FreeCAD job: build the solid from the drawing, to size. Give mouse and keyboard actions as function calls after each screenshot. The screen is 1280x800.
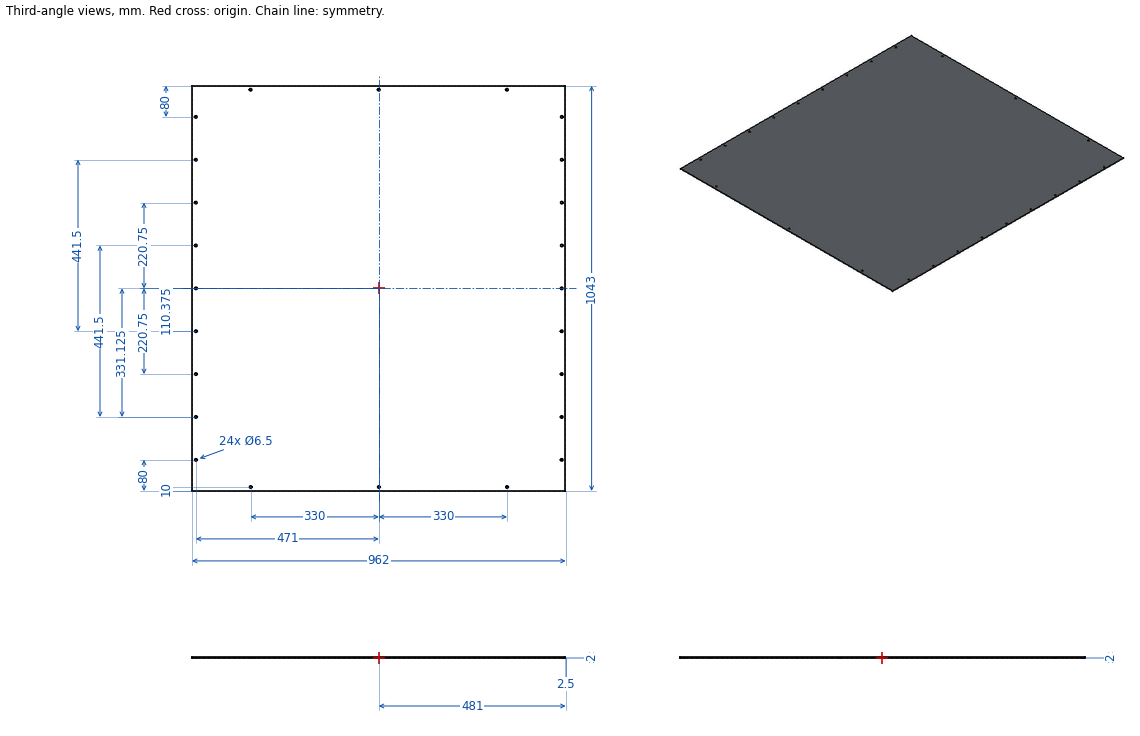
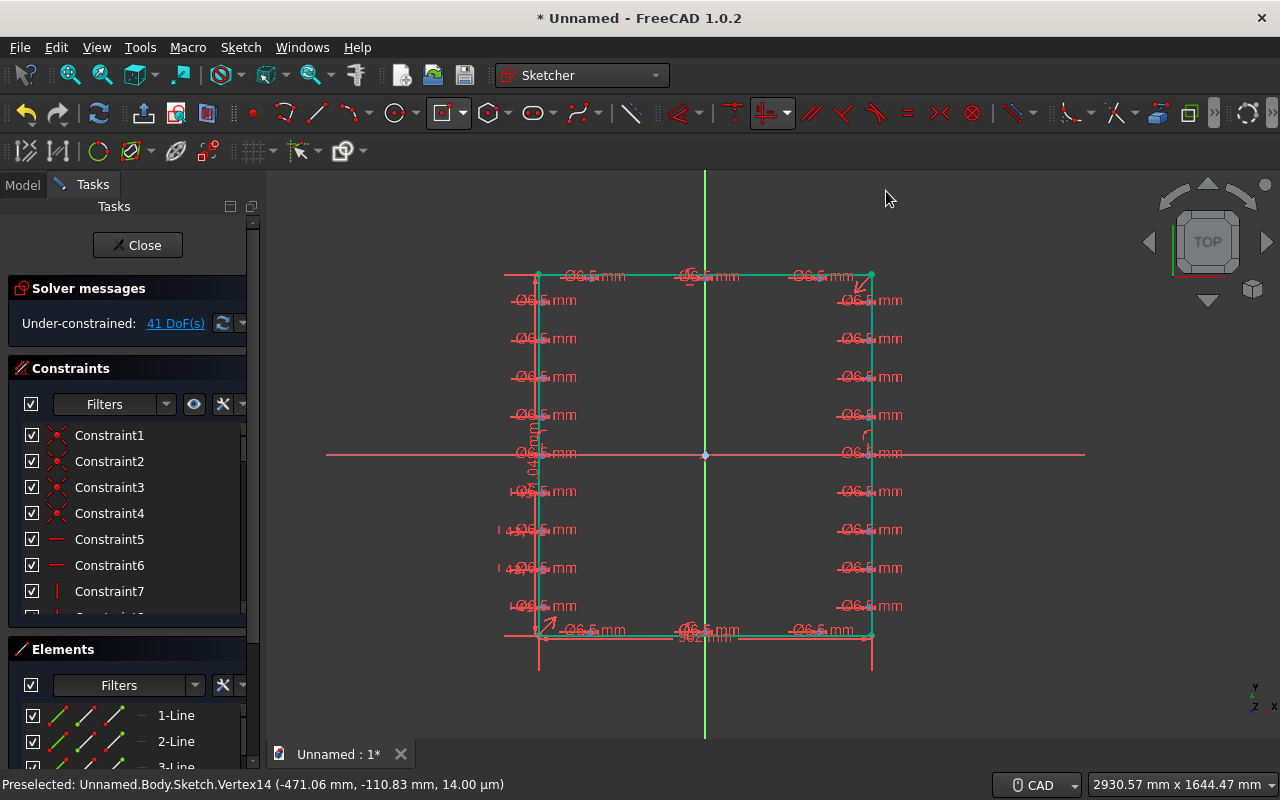
click(591, 632)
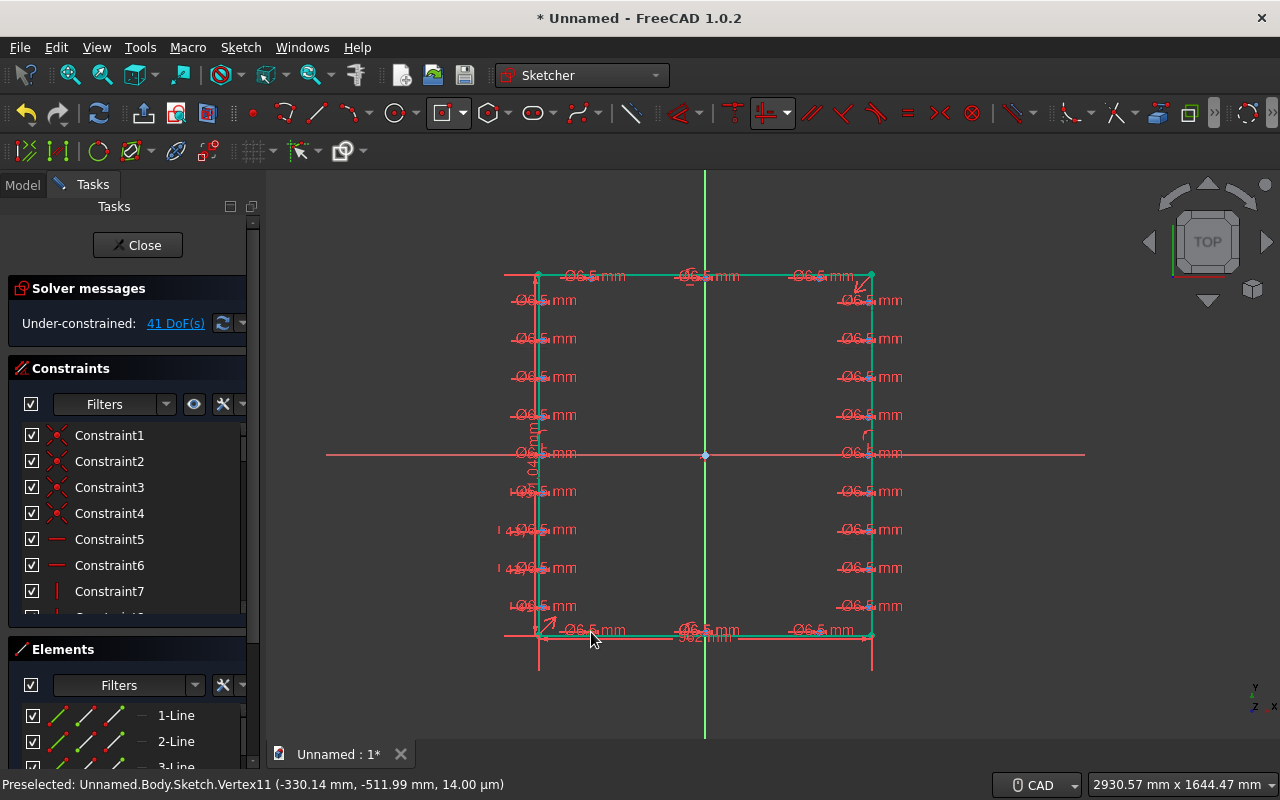
click(705, 632)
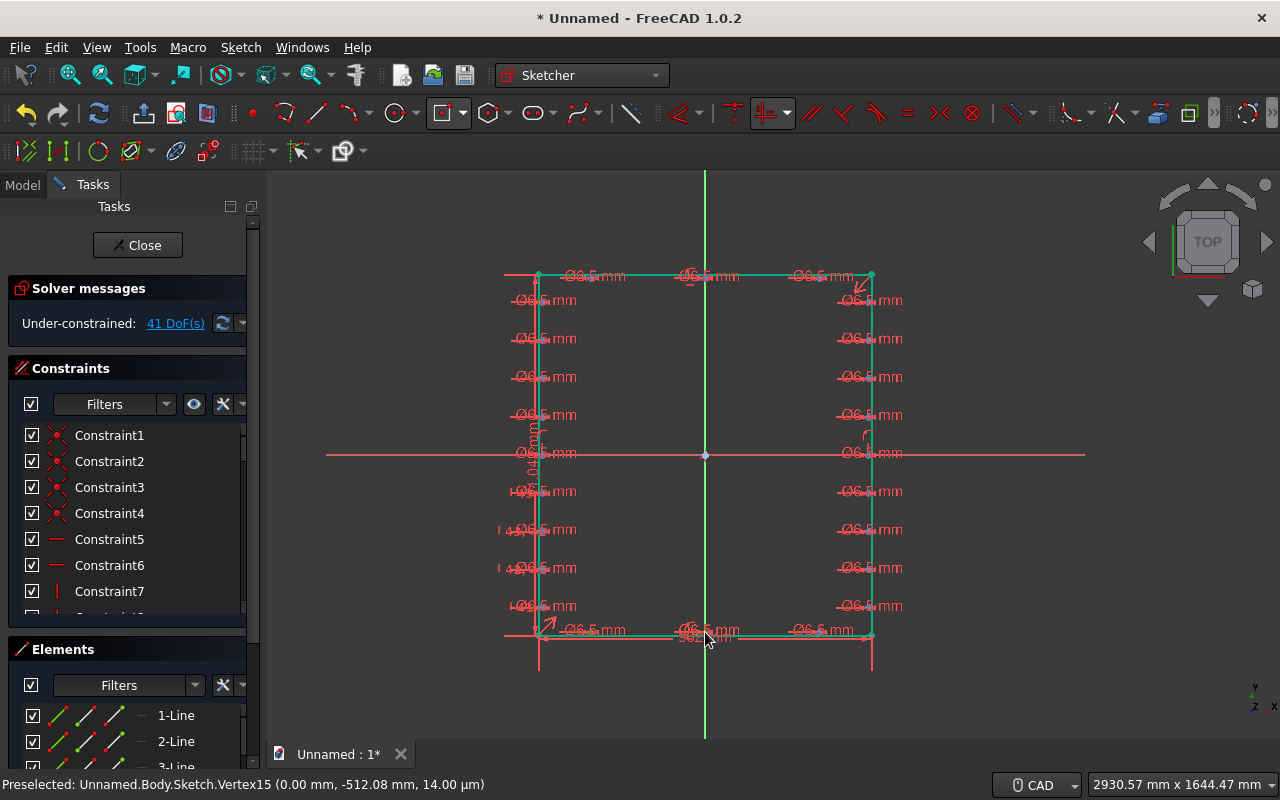
click(790, 114)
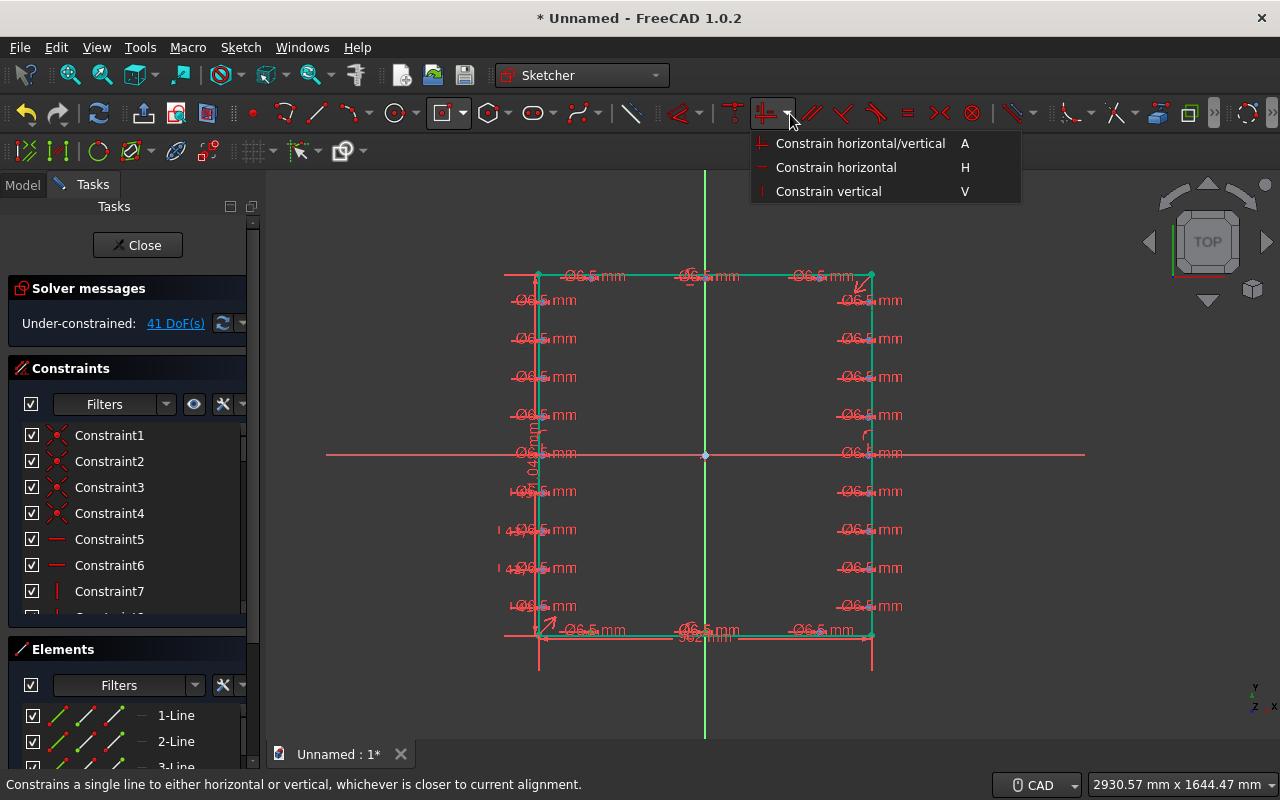
click(886, 167)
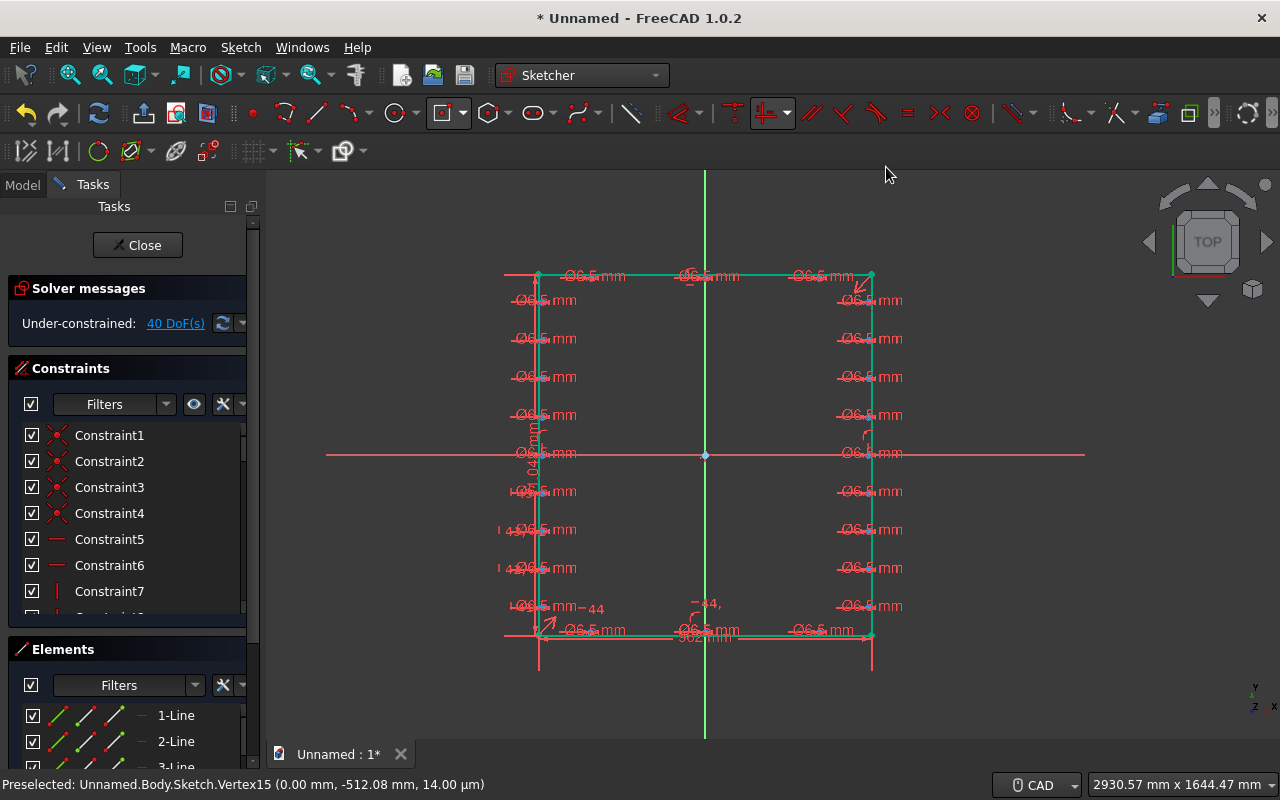
click(705, 632)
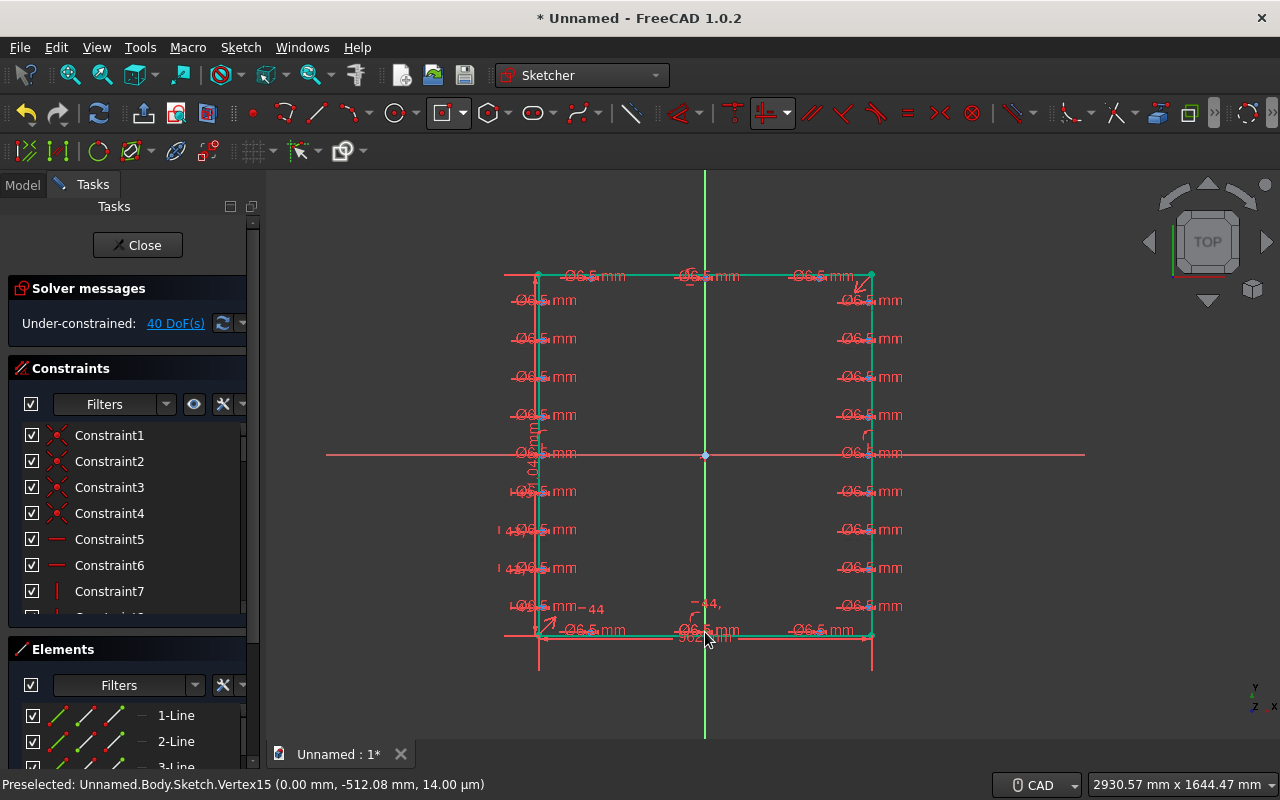
click(819, 632)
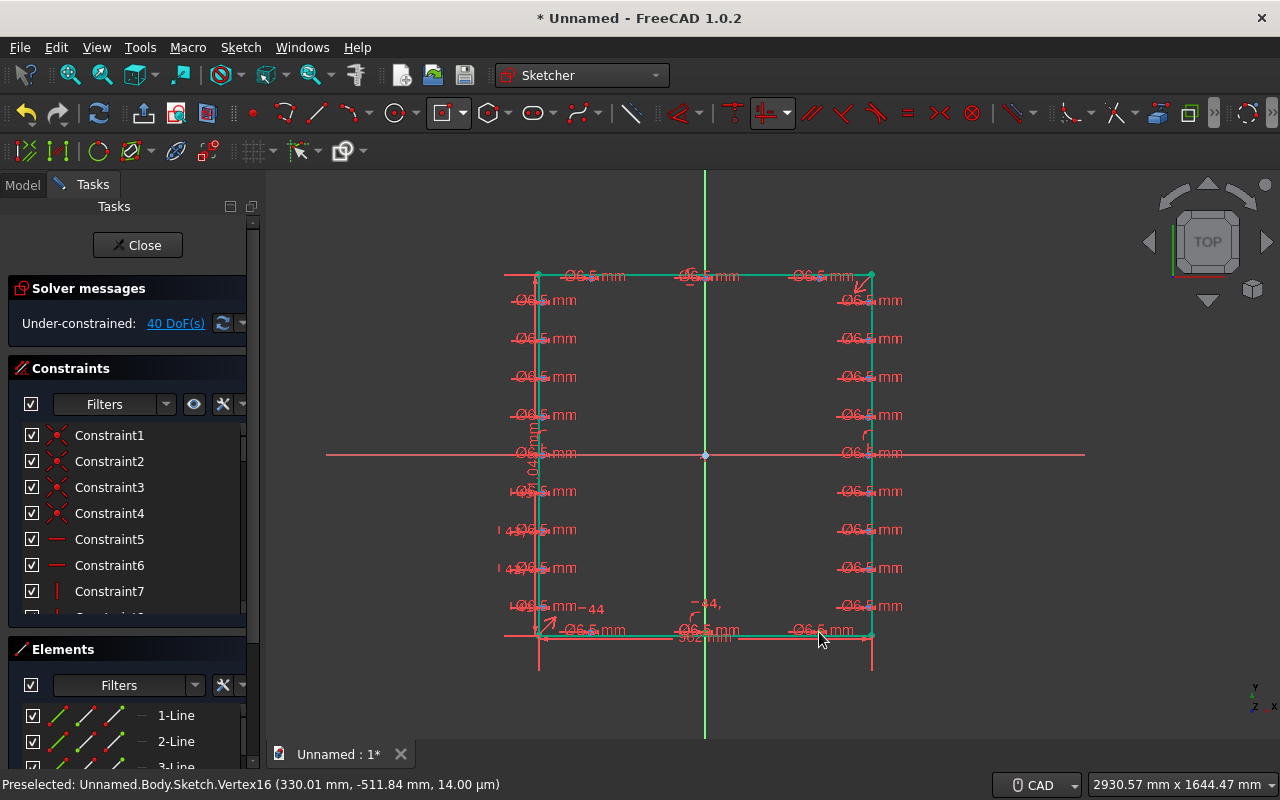
key(h)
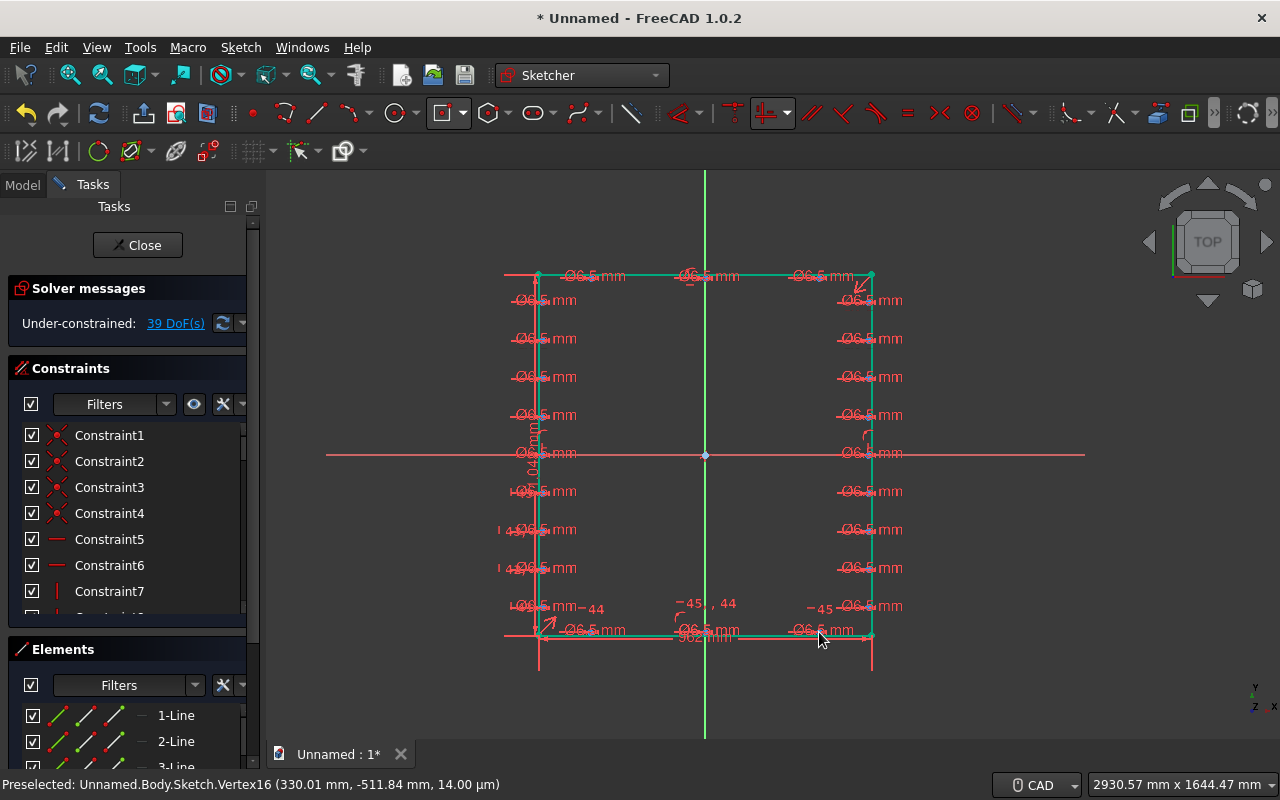
click(542, 608)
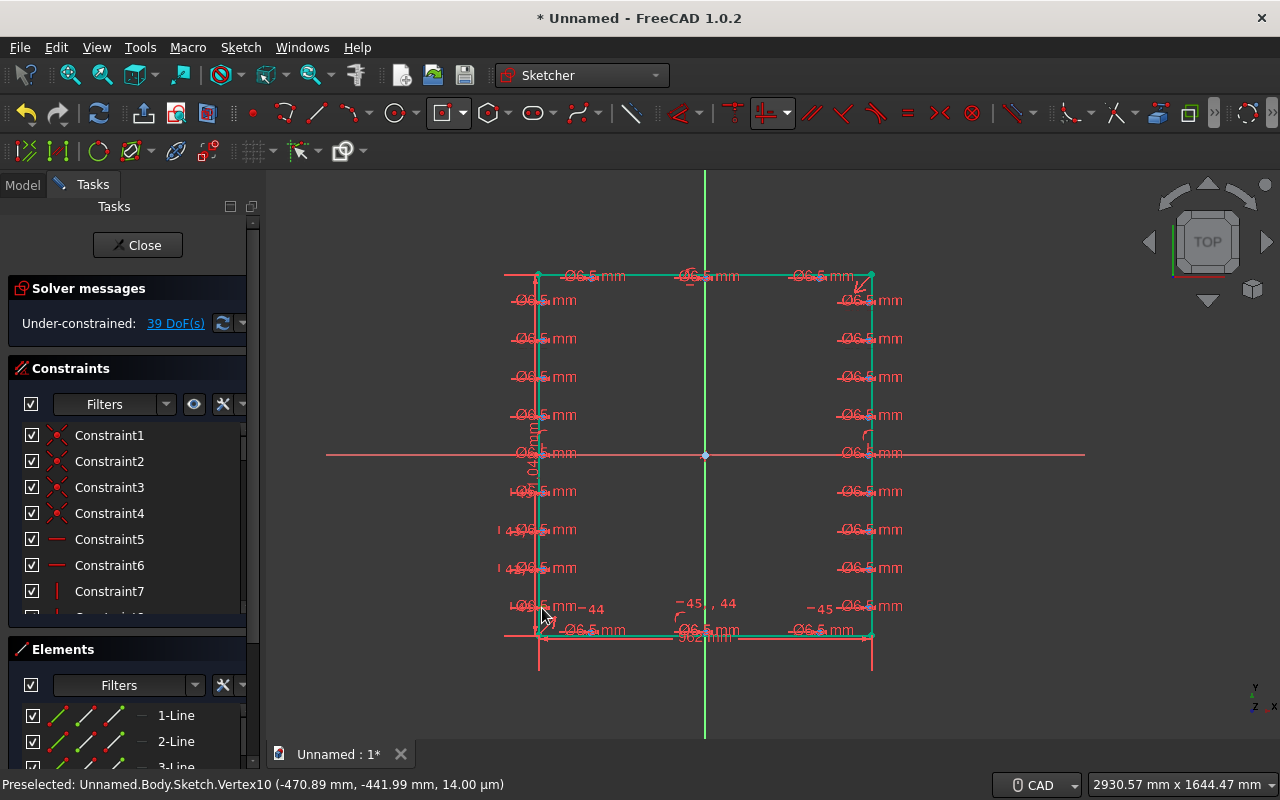
click(868, 608)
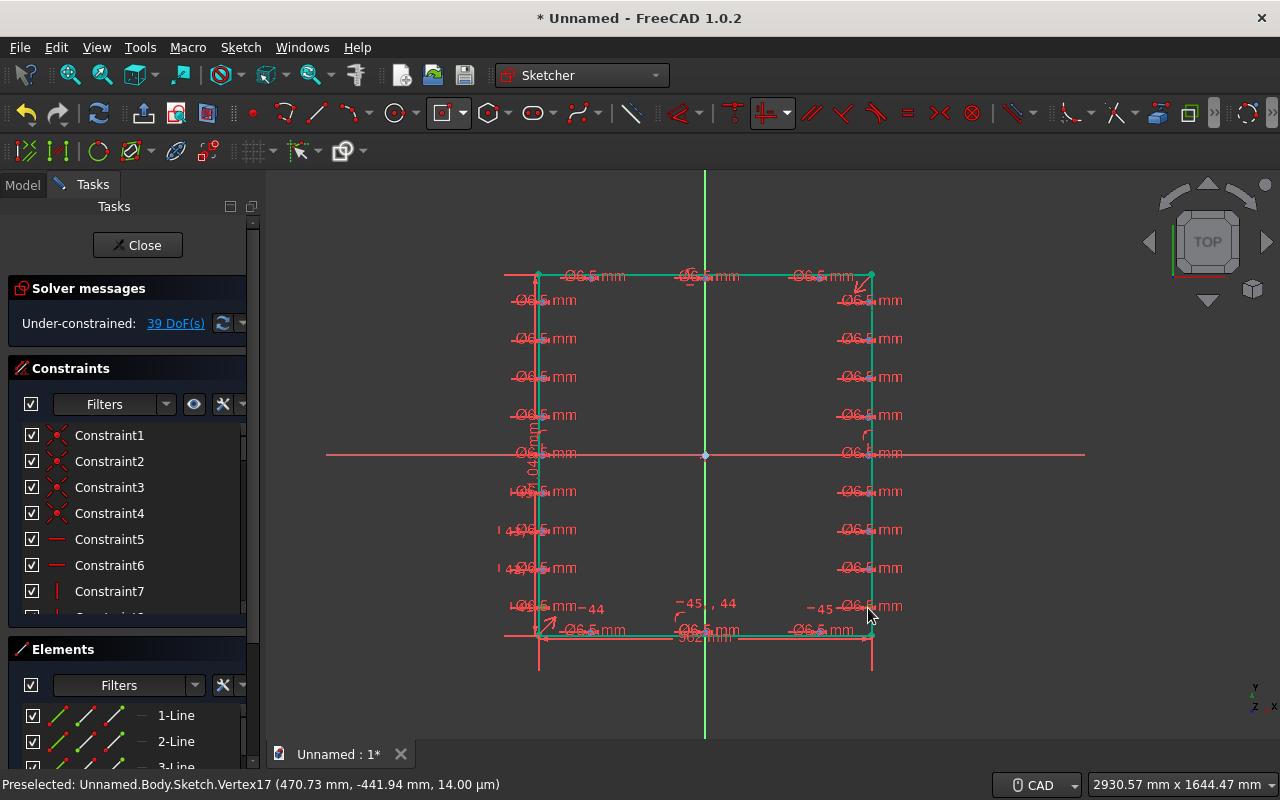
click(790, 114)